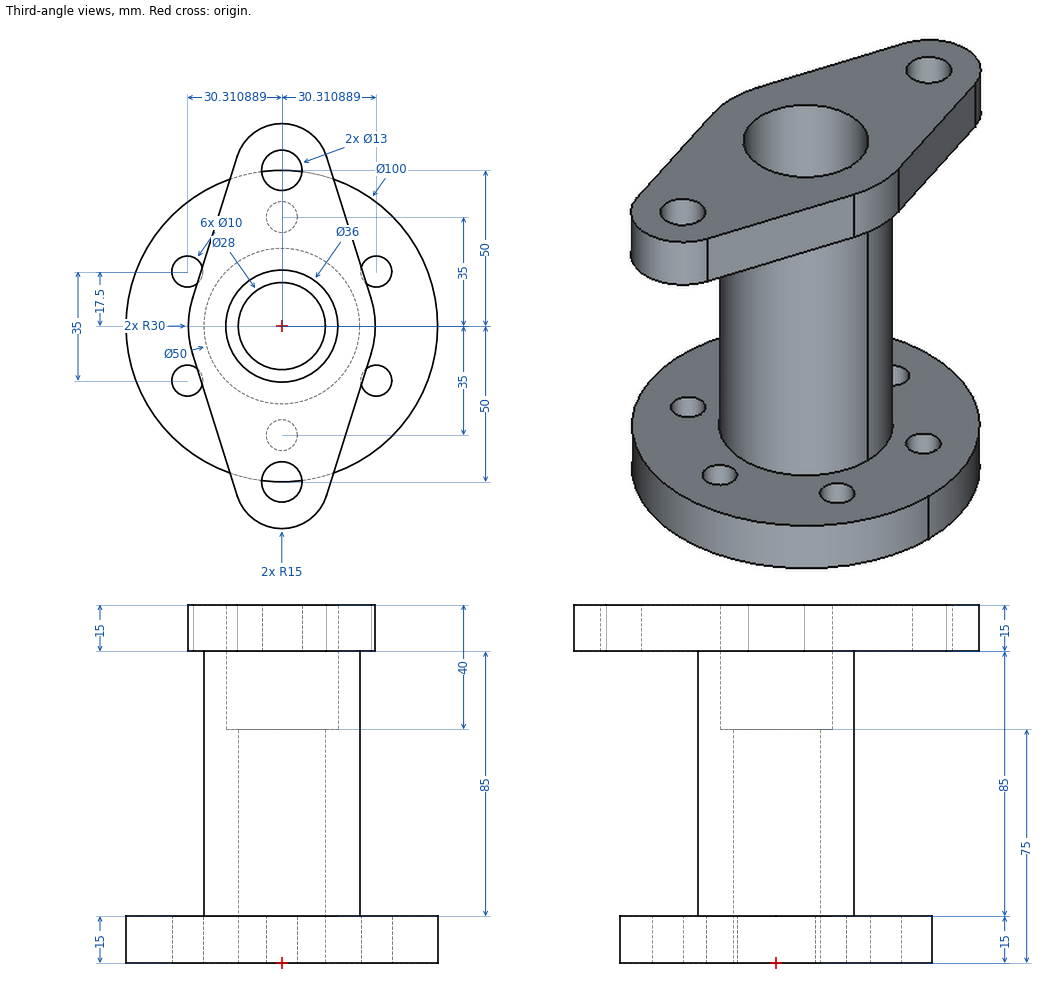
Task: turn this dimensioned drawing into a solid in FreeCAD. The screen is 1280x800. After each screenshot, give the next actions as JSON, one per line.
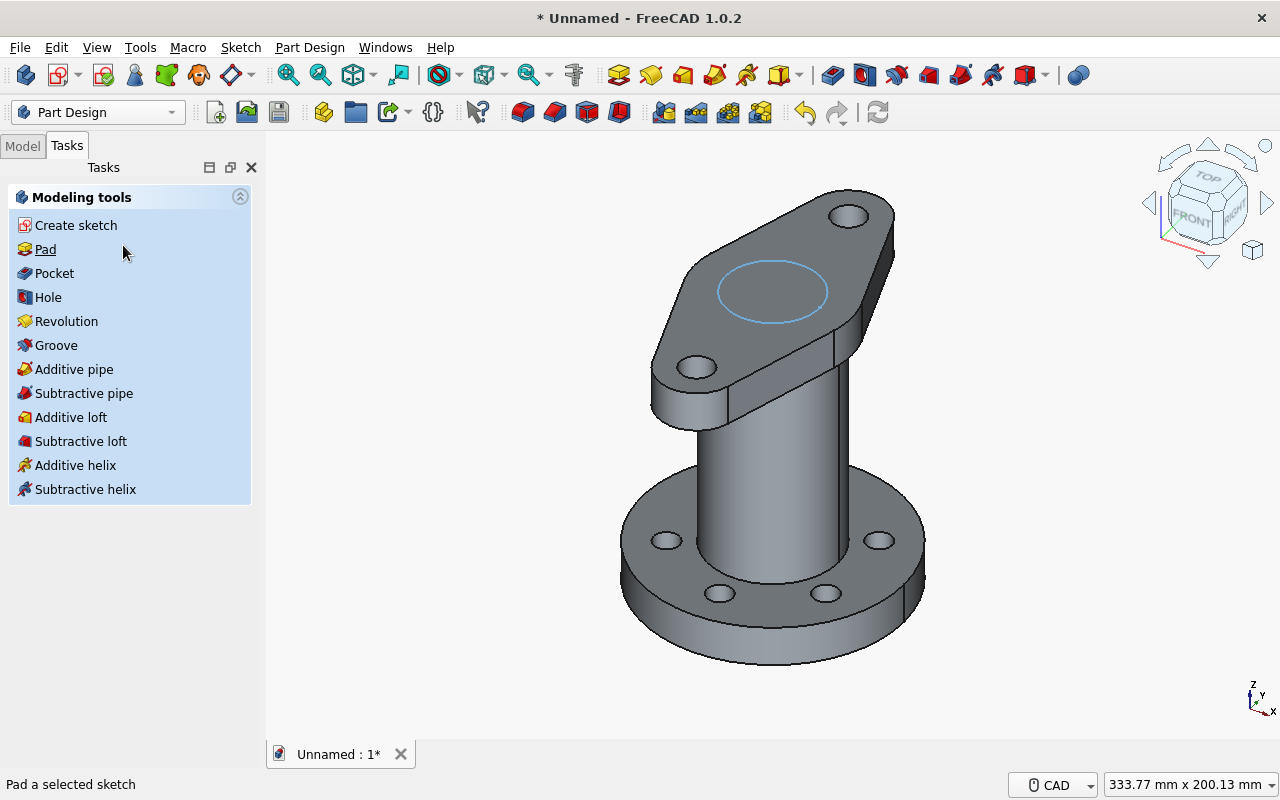
{"action": "left_click", "coordinate": [834, 76]}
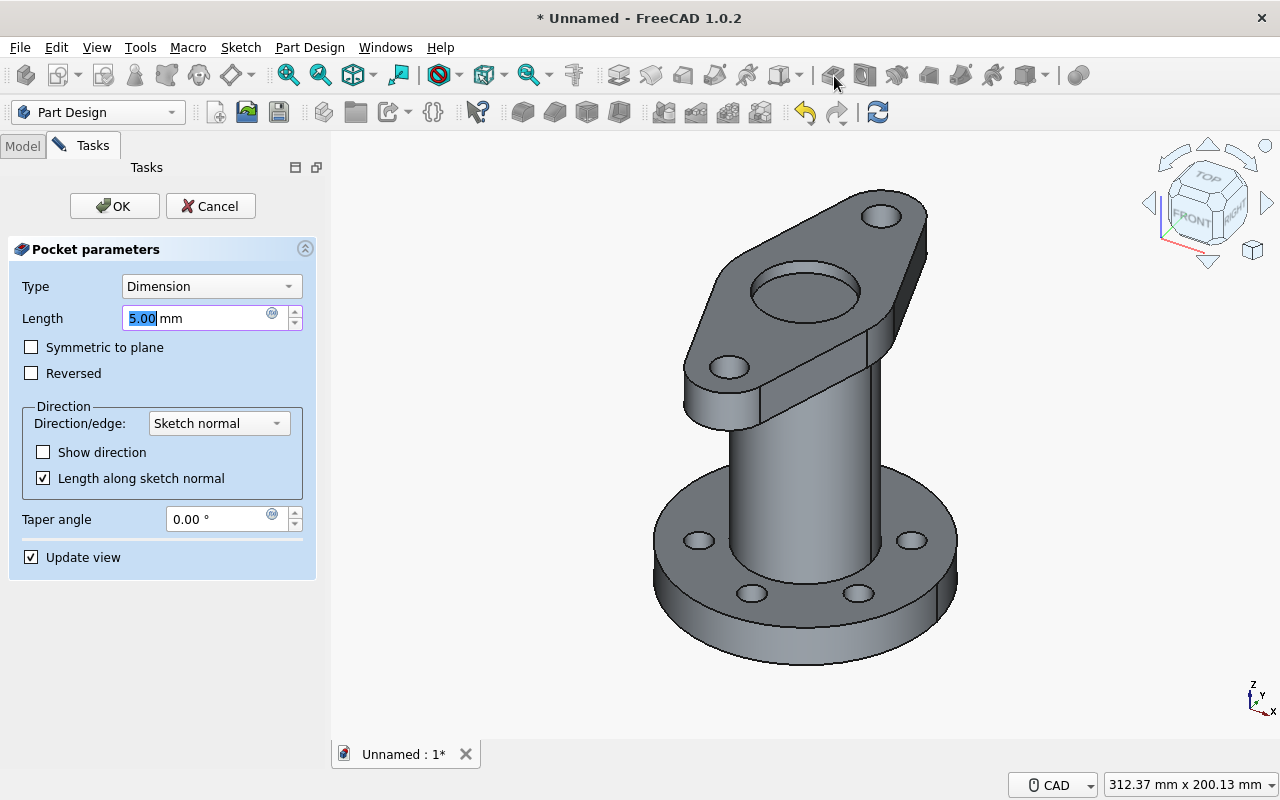
{"action": "type", "text": "40"}
{"action": "key", "text": "Tab"}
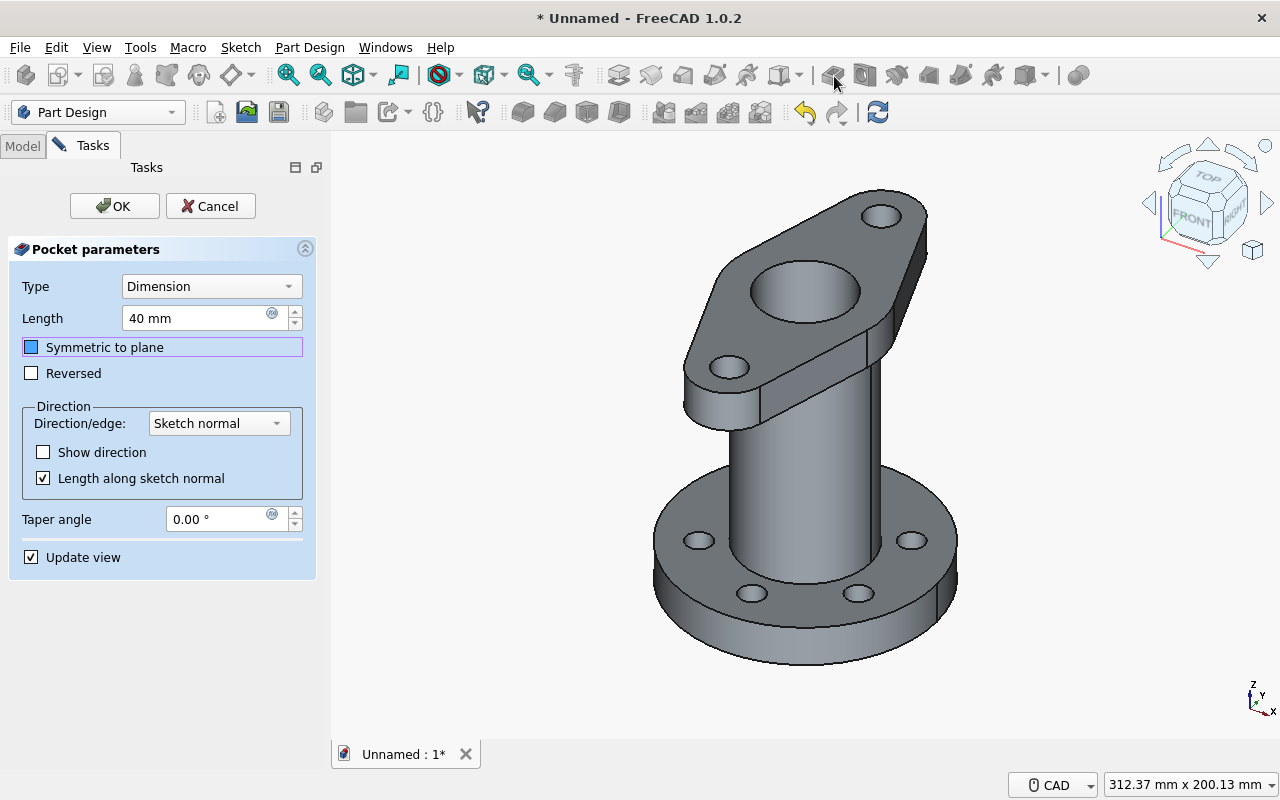
{"action": "left_click", "coordinate": [115, 206]}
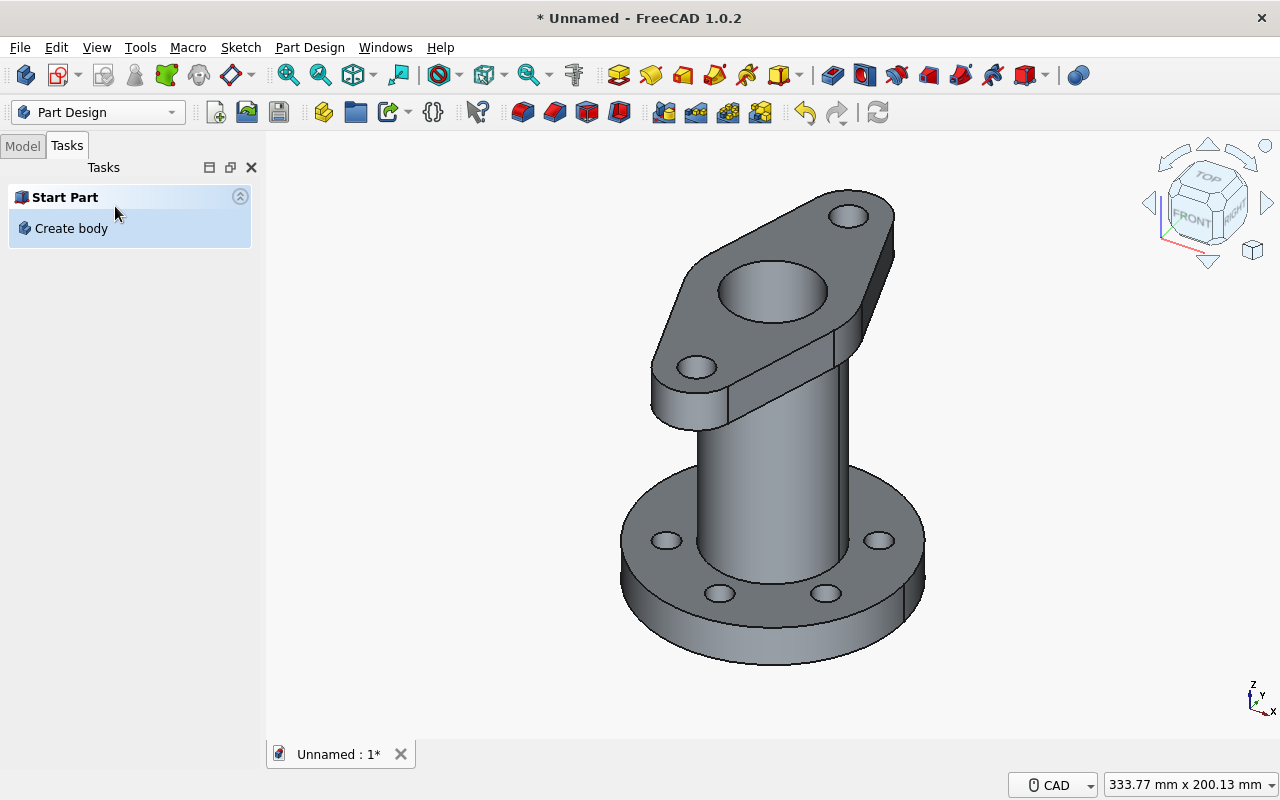
{"action": "key", "text": "0"}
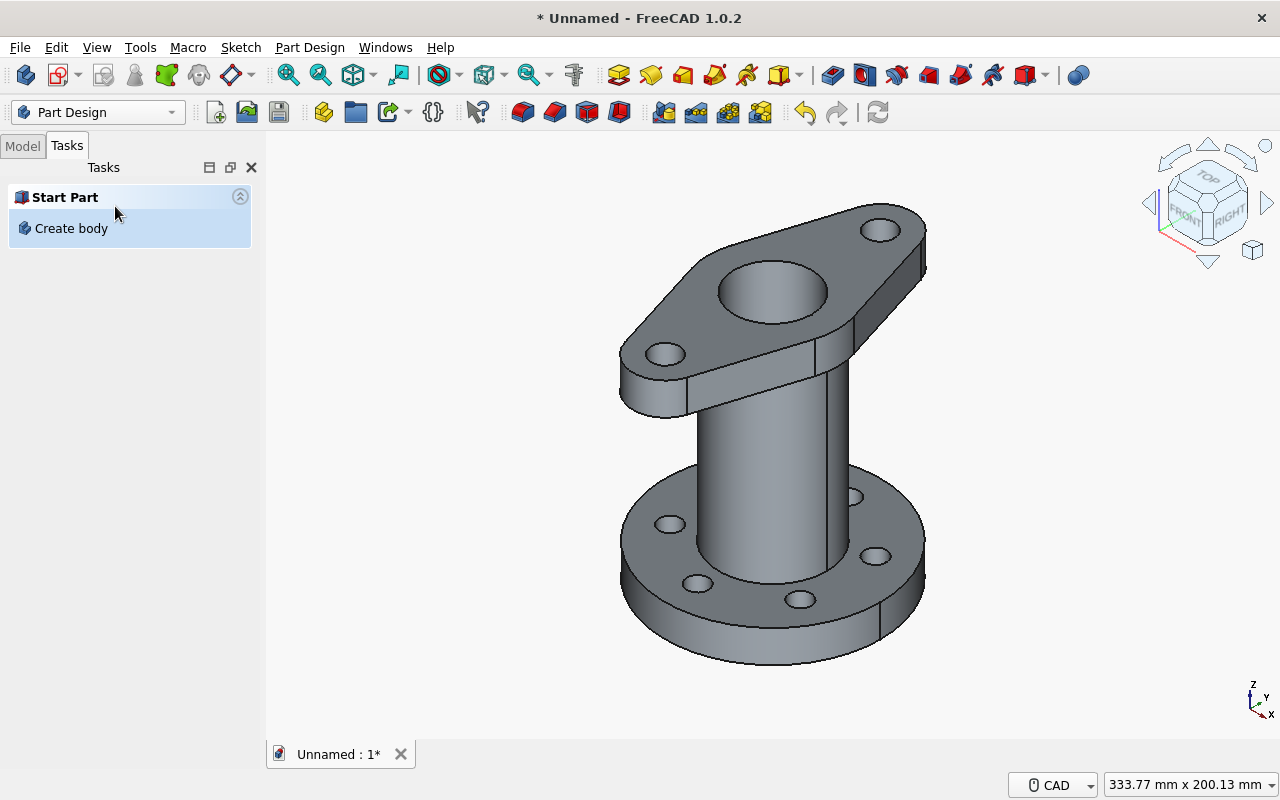
{"action": "key", "text": "2"}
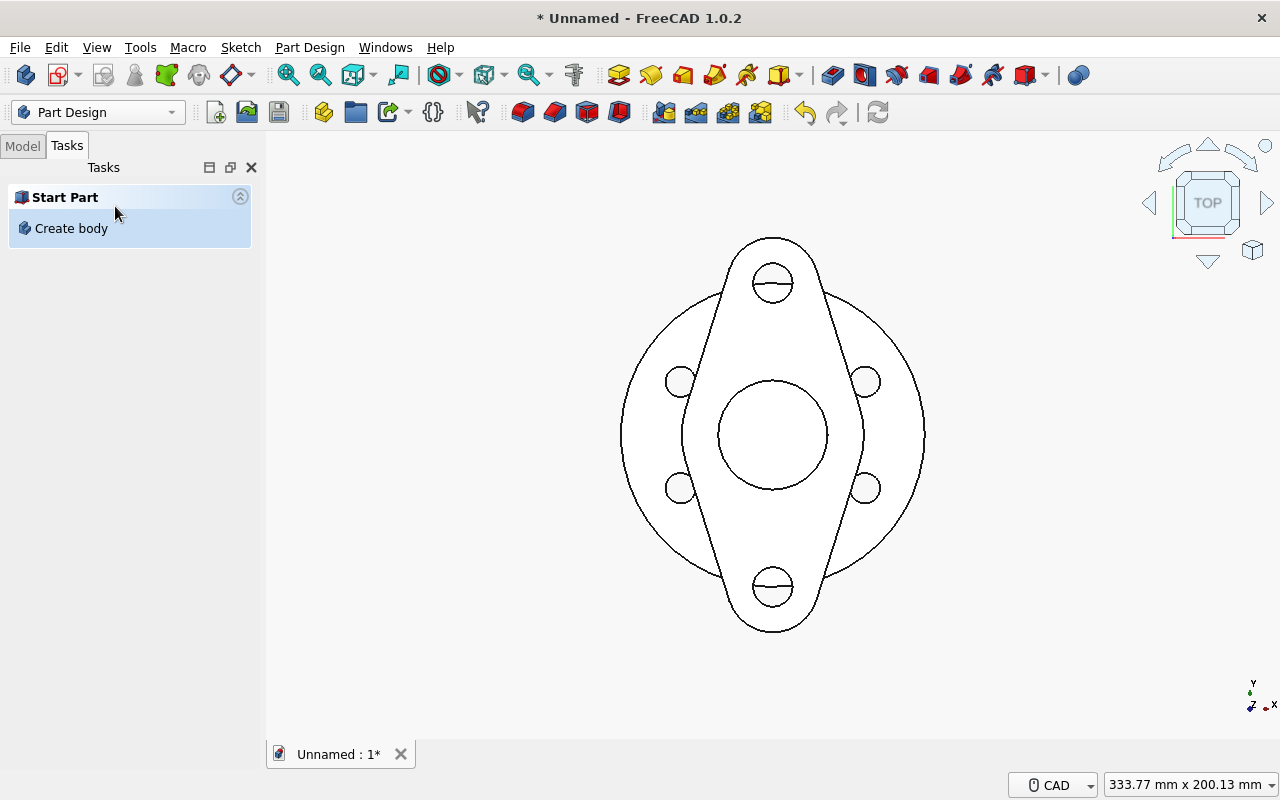
{"action": "left_click", "coordinate": [773, 434]}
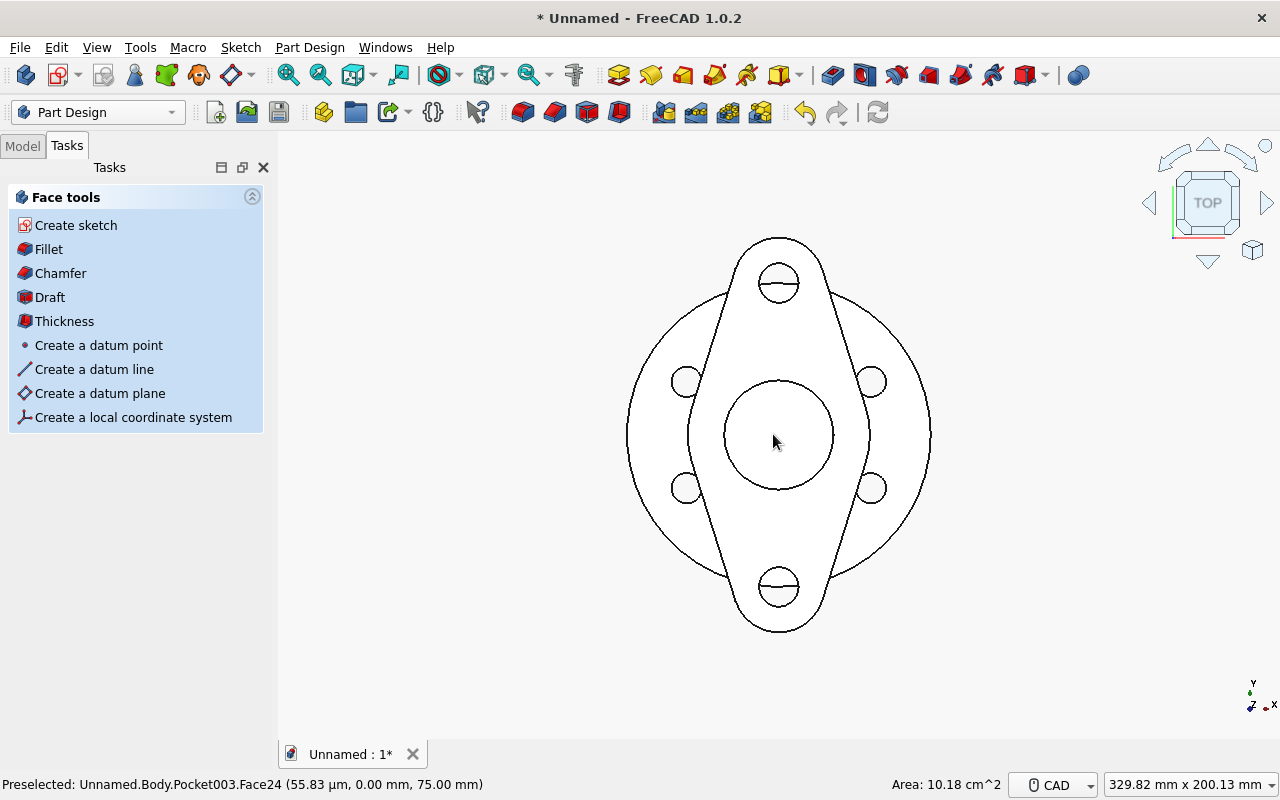
{"action": "left_click", "coordinate": [58, 76]}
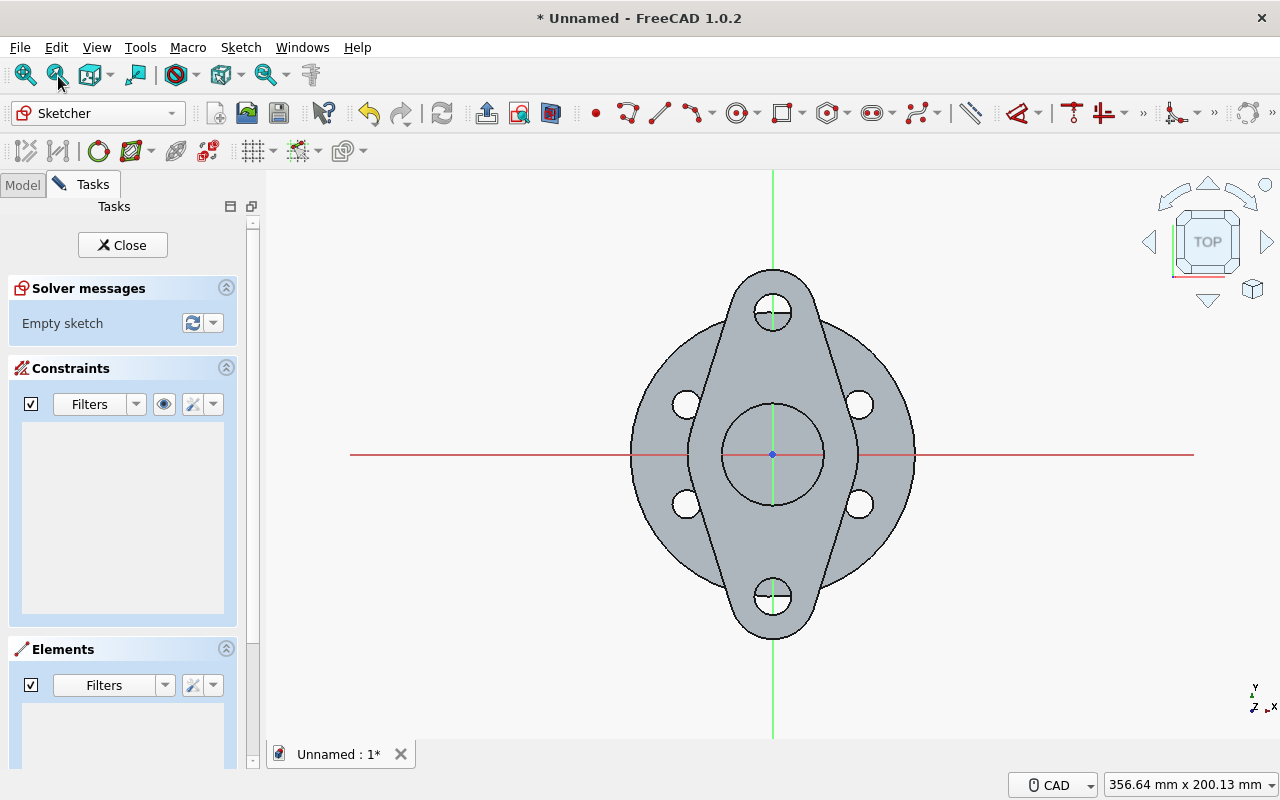
{"action": "scroll", "coordinate": [790, 454], "scroll_direction": "up", "scroll_amount": 8}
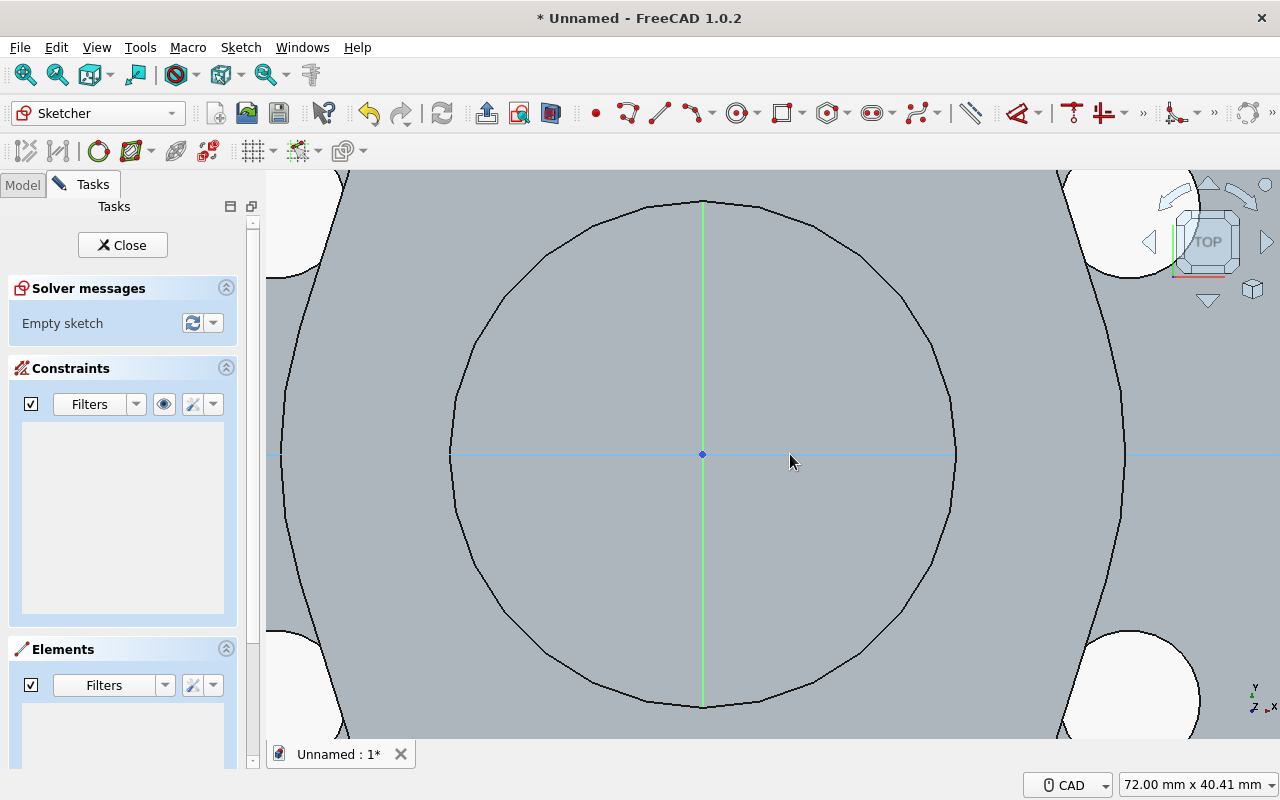
{"action": "key", "text": "g c"}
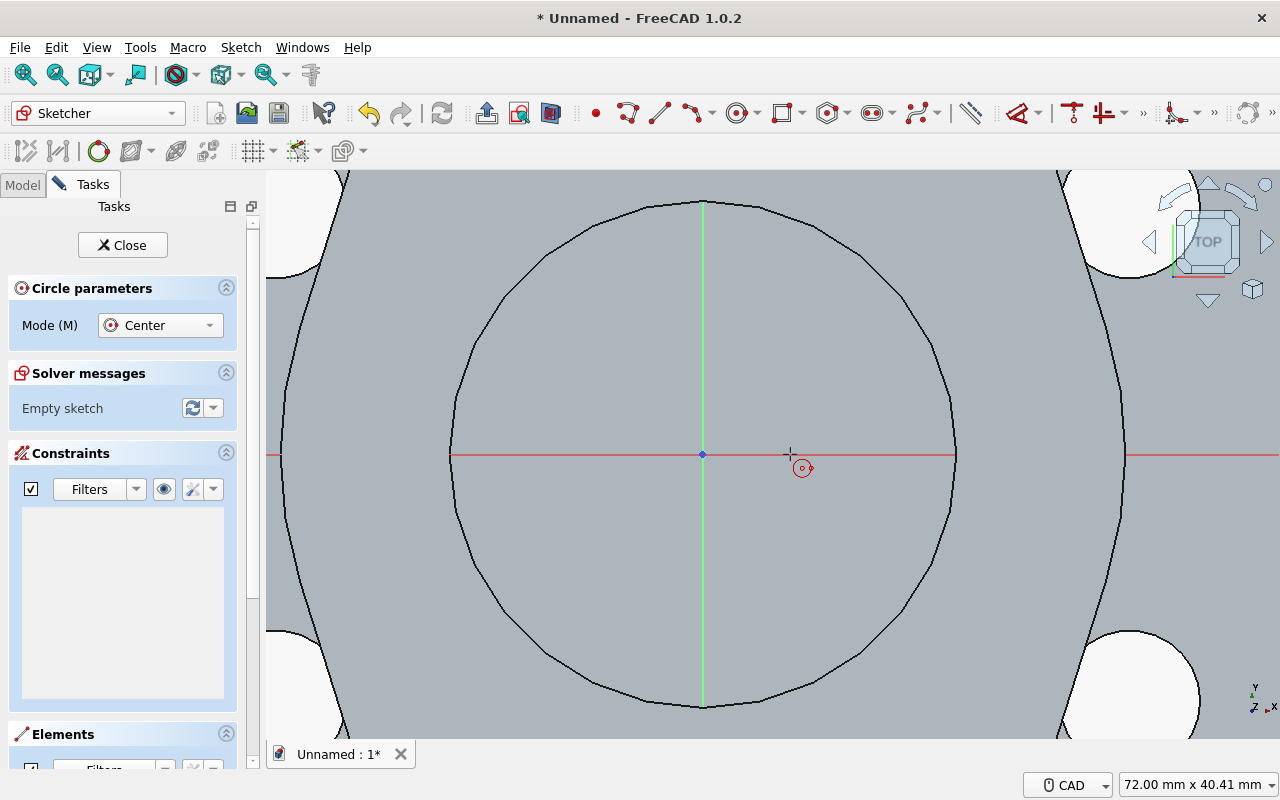
{"action": "left_click", "coordinate": [703, 454]}
{"action": "mouse_move", "coordinate": [842, 315]}